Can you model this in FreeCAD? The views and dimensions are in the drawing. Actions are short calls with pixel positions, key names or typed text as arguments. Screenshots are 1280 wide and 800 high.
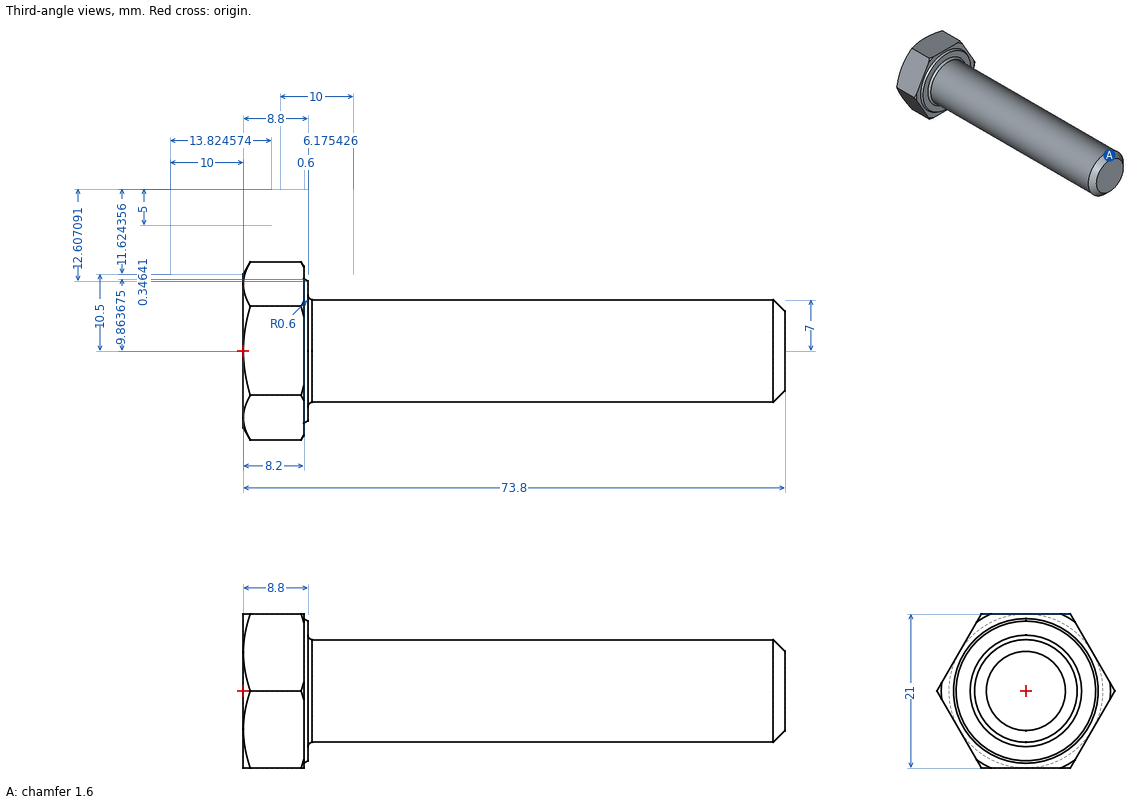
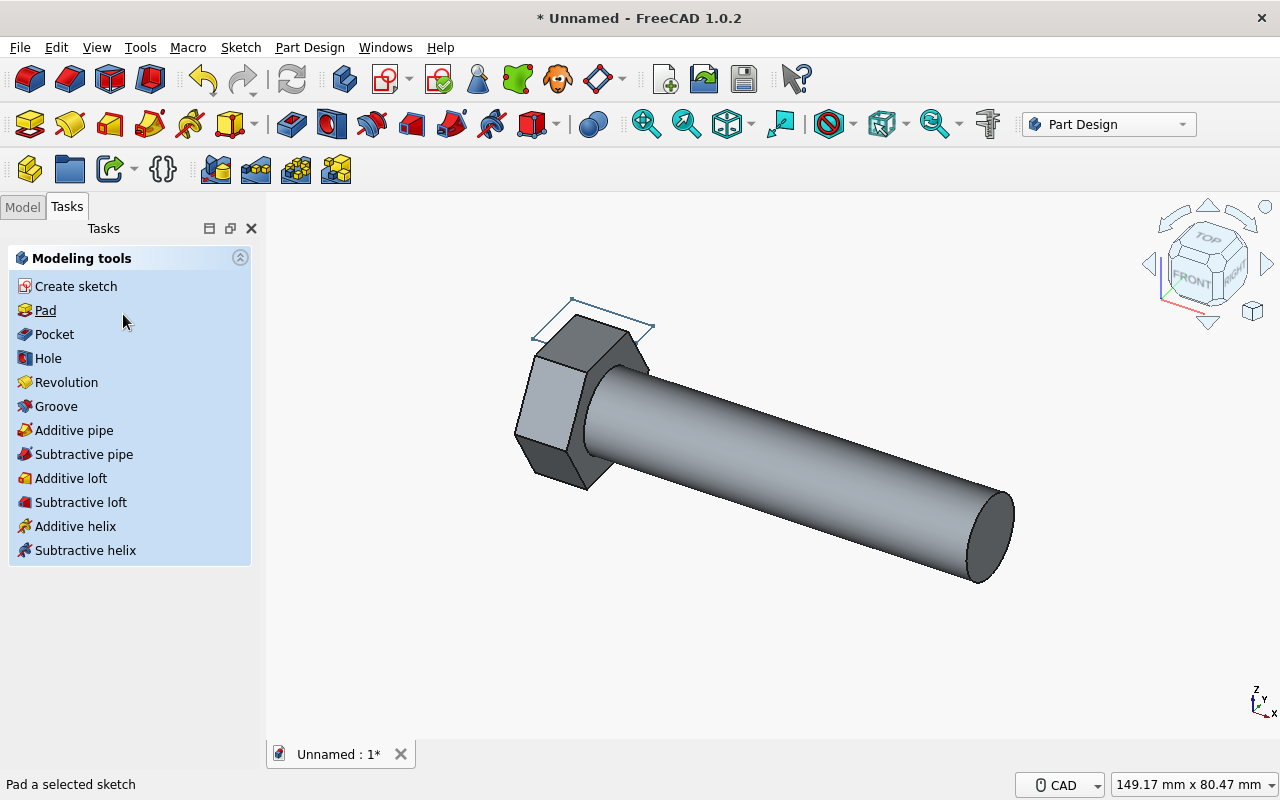
click(372, 124)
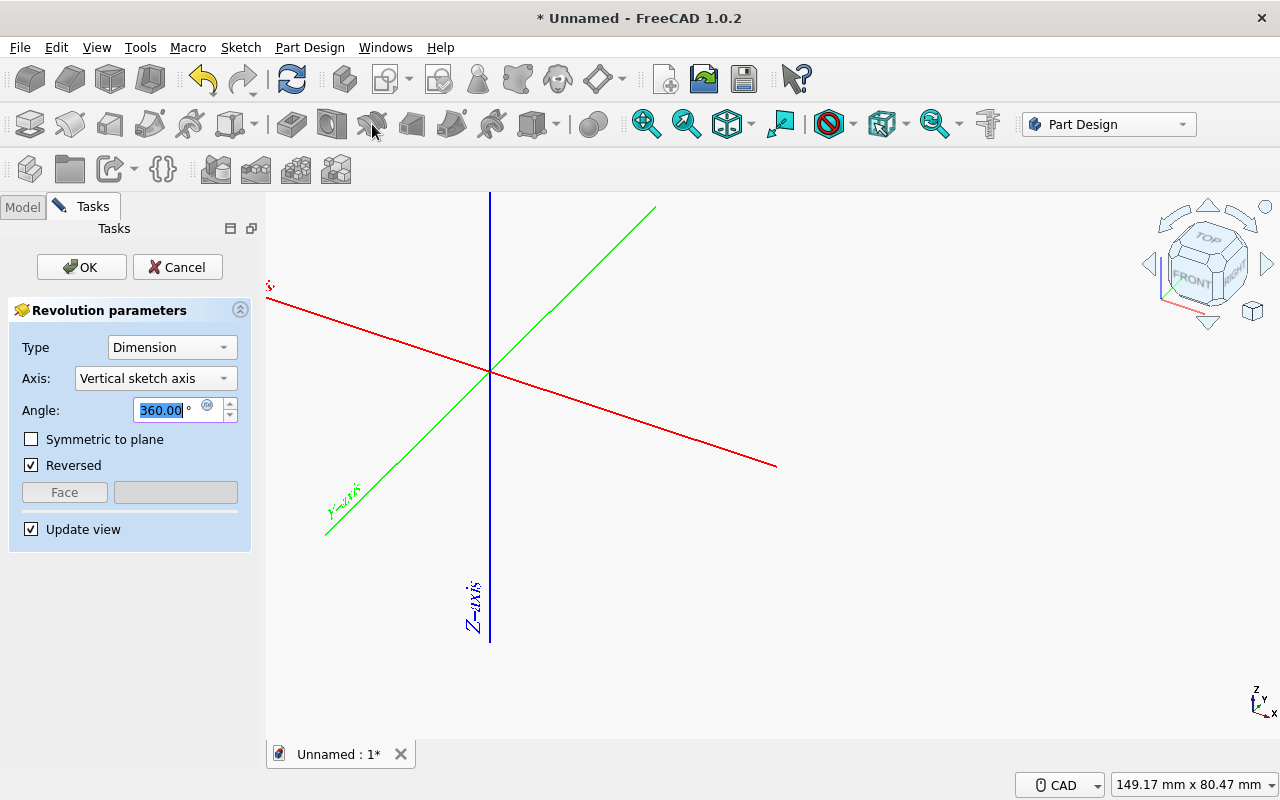
click(156, 378)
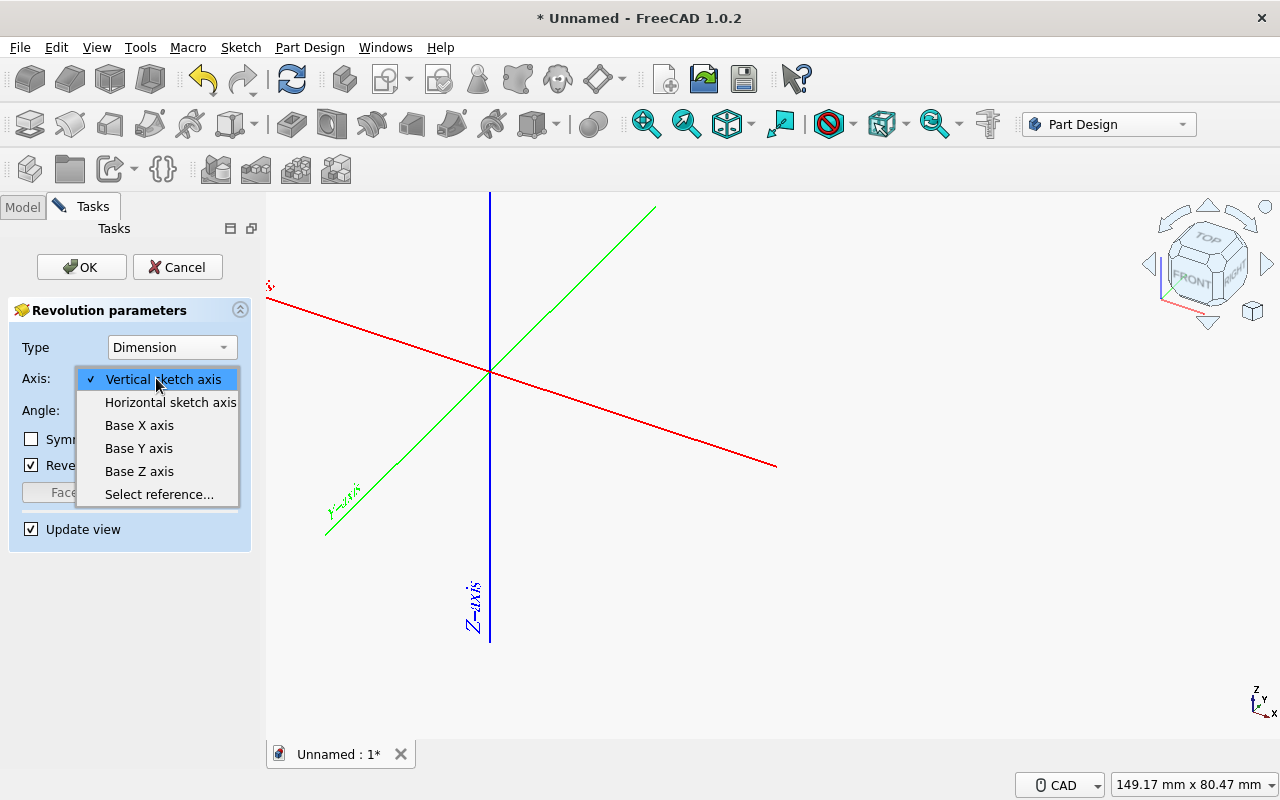
click(156, 402)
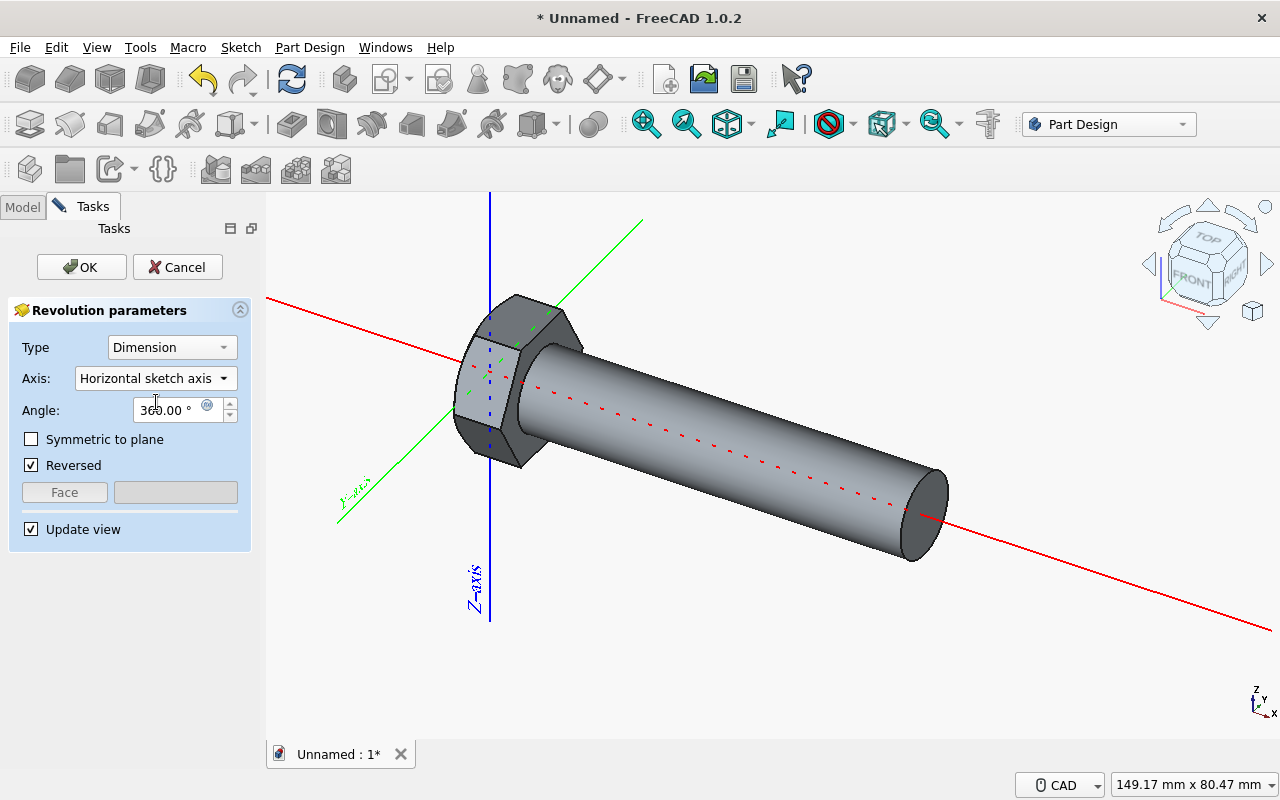
click(82, 267)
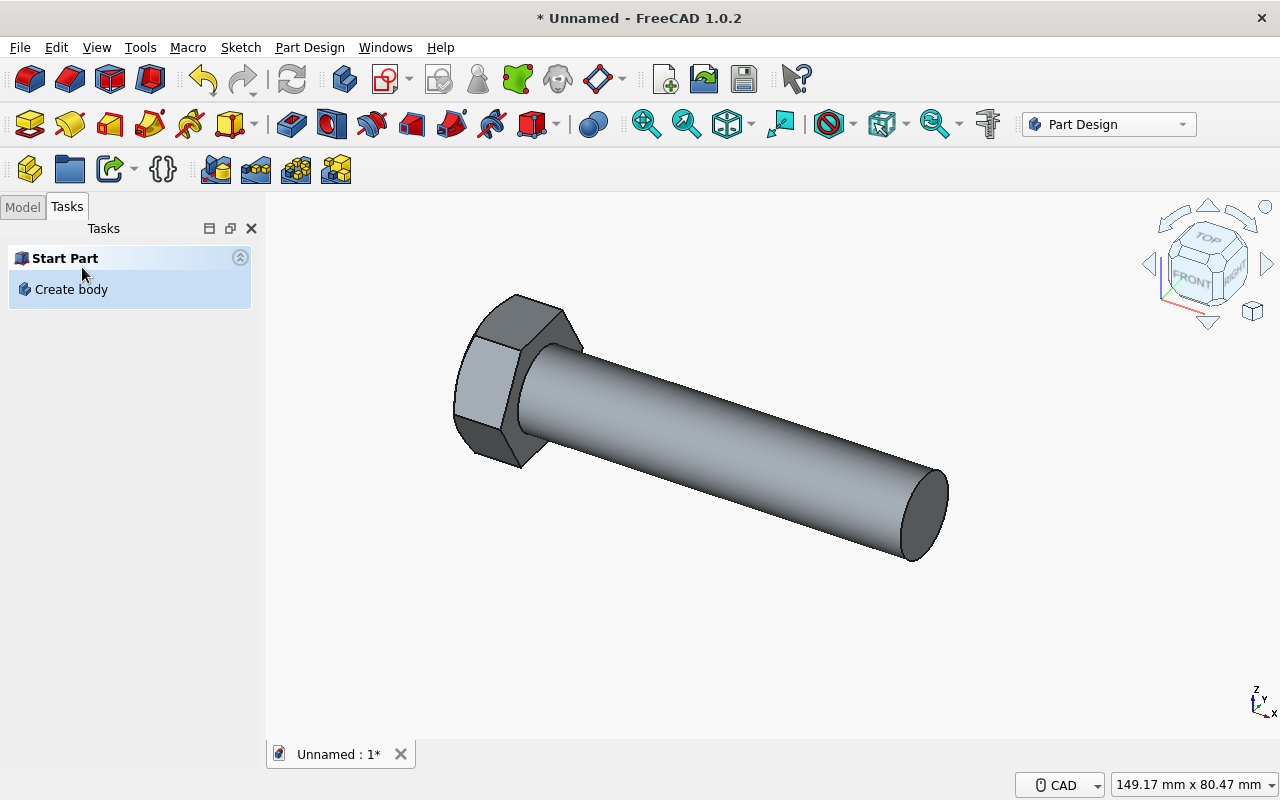
click(386, 80)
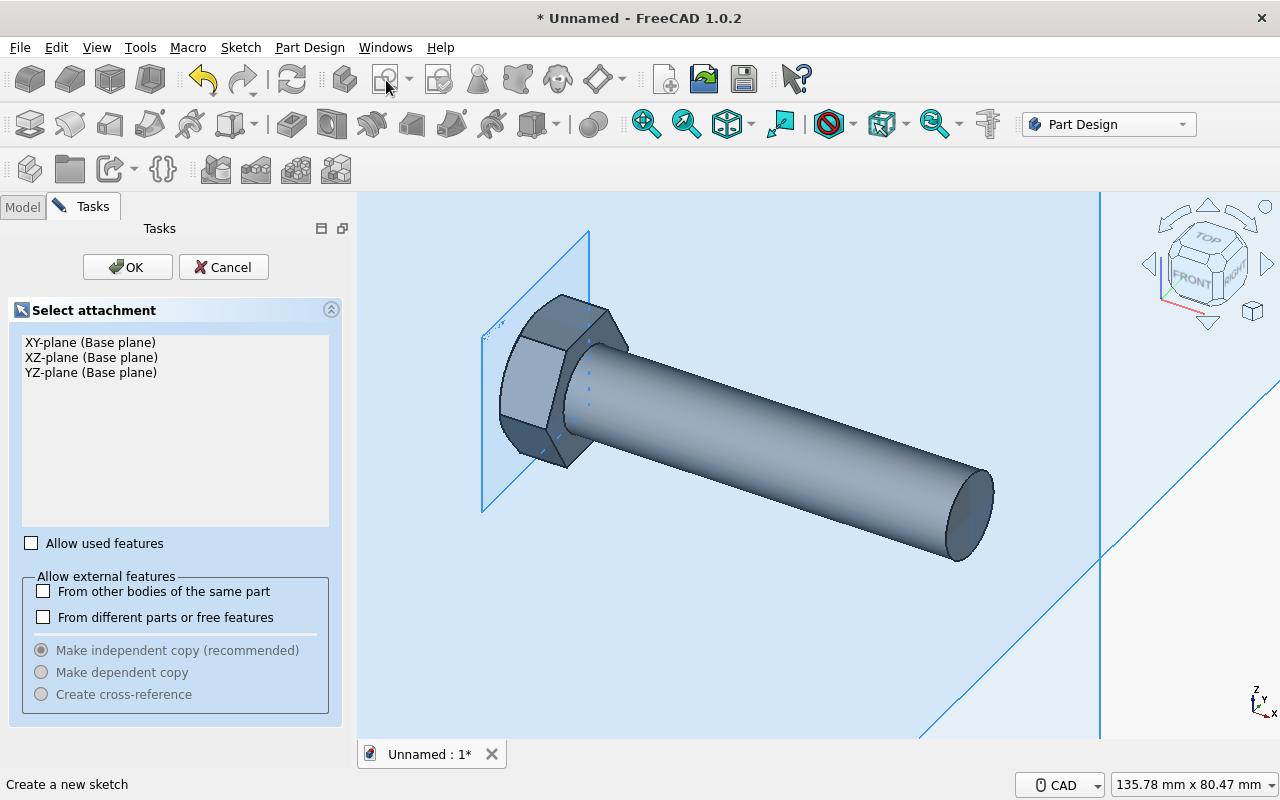
click(82, 342)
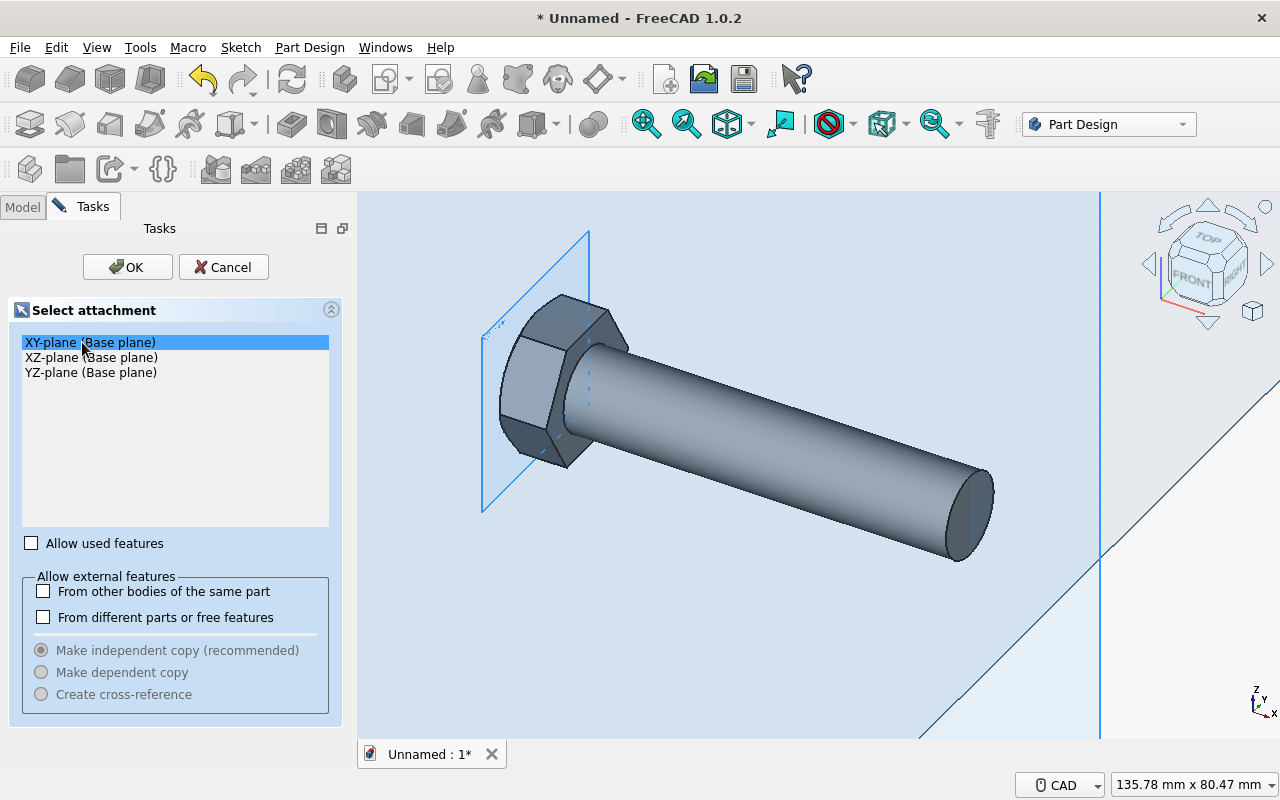
click(128, 267)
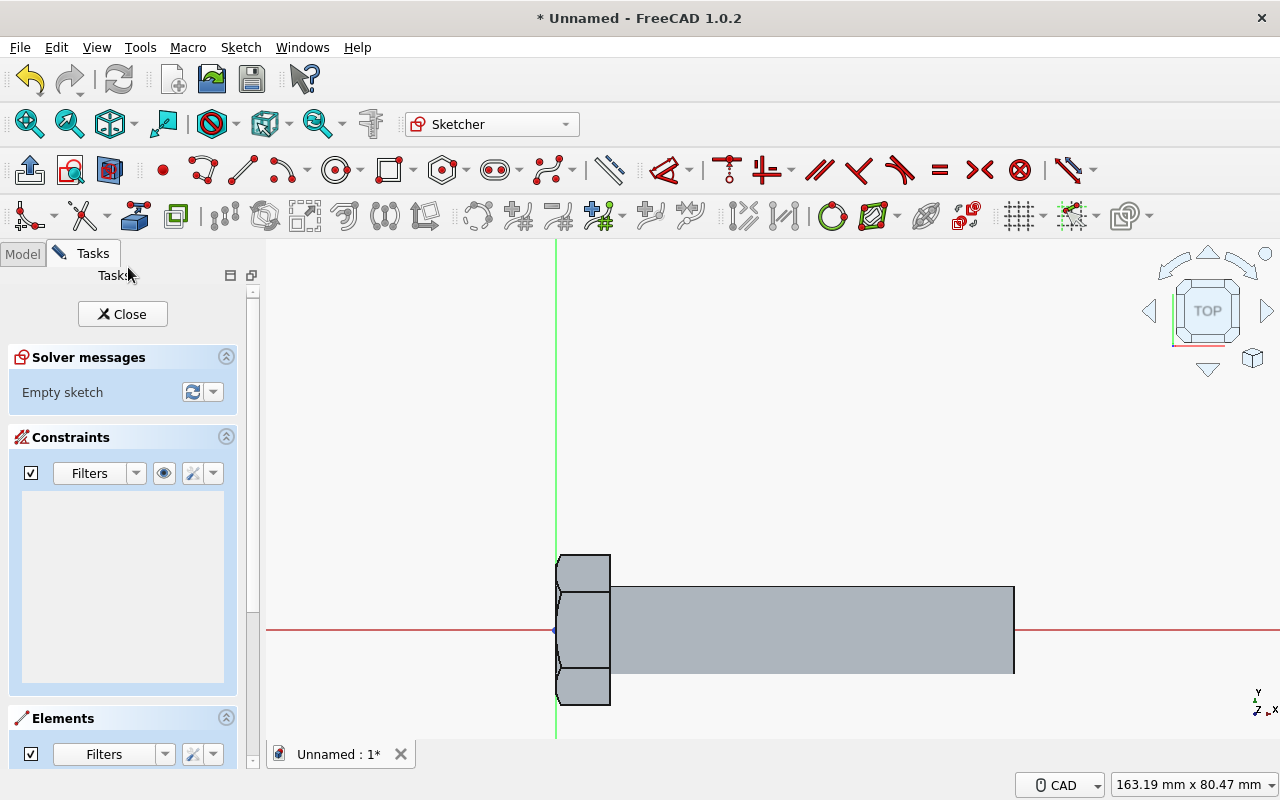
click(110, 170)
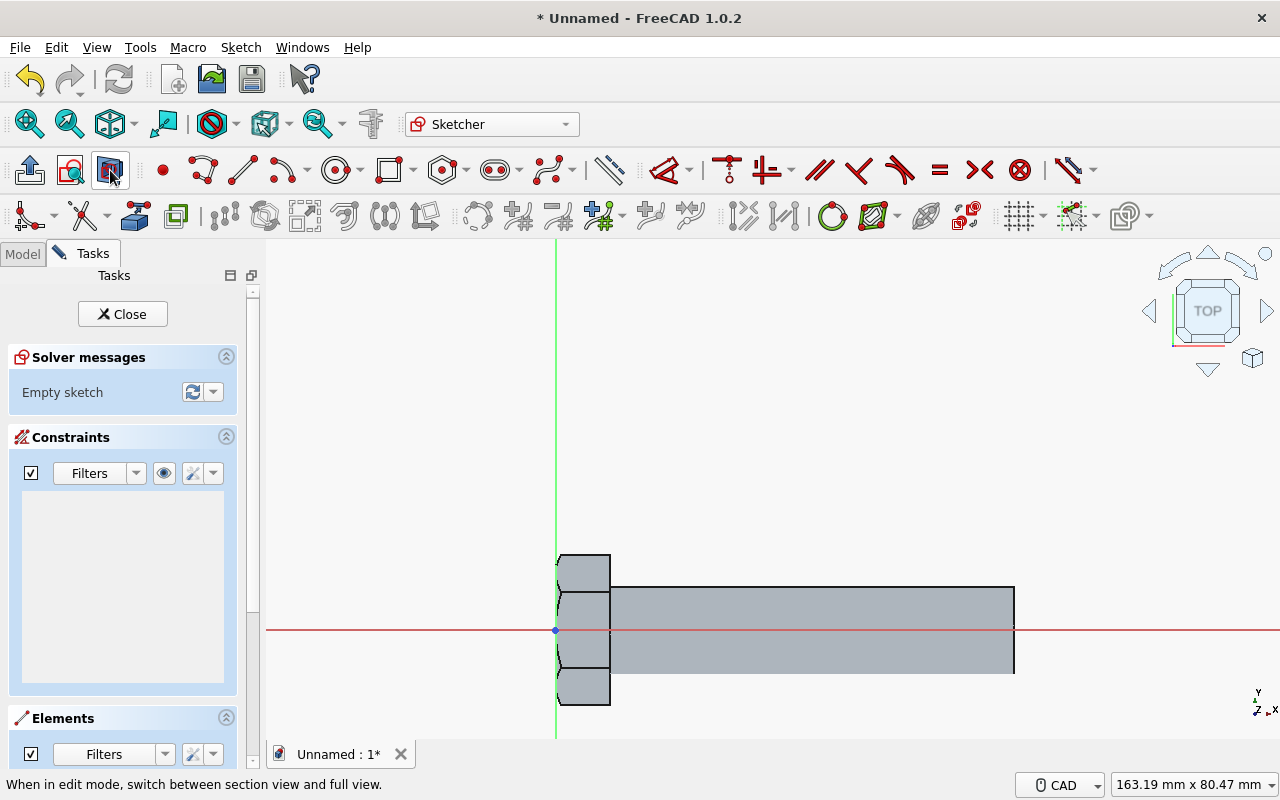
scroll(519, 620, up, 4)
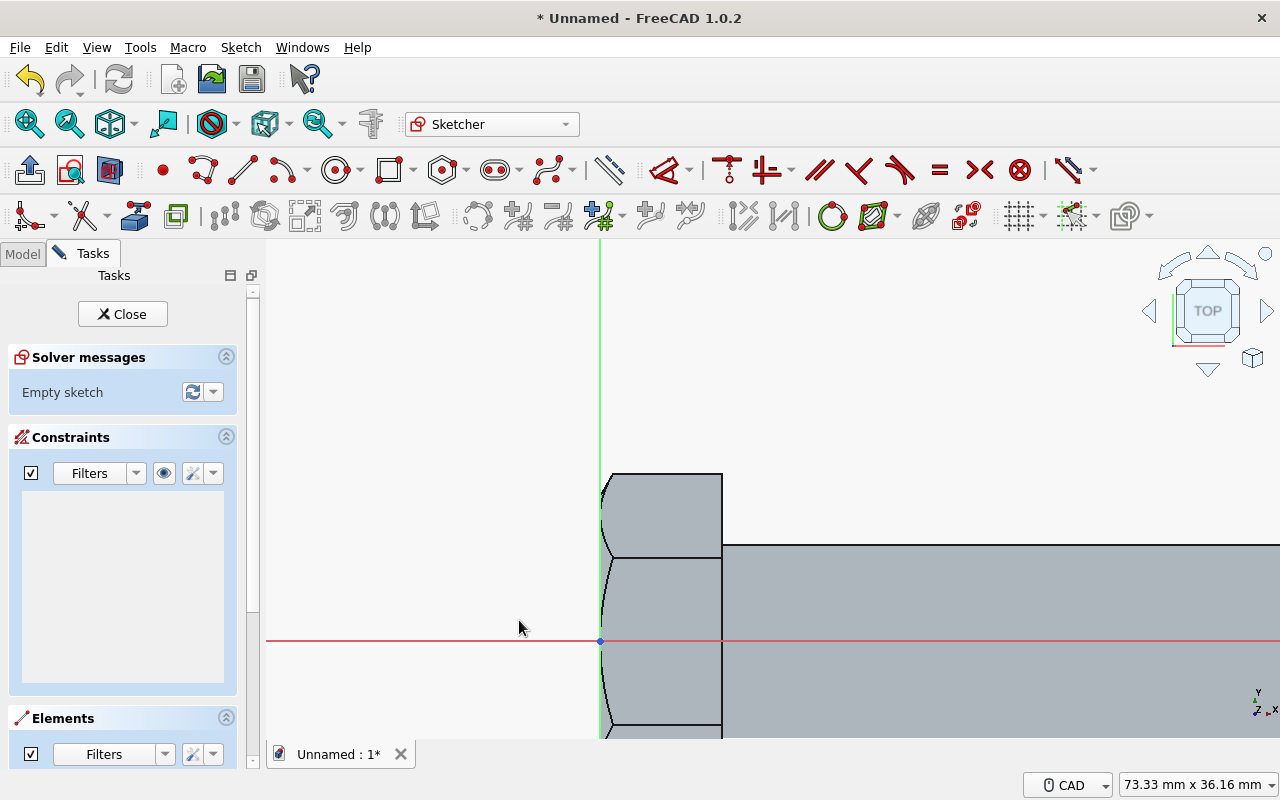
click(204, 170)